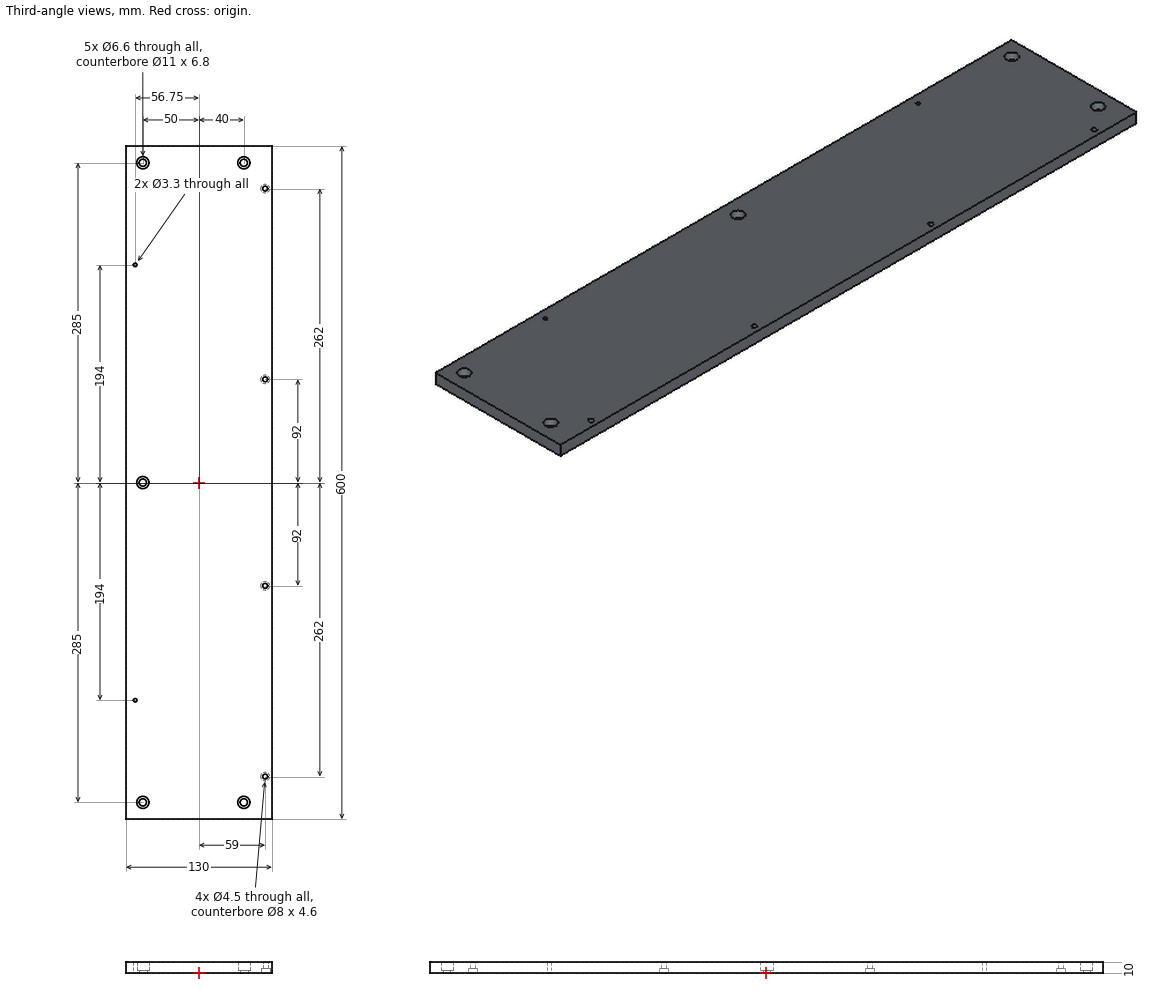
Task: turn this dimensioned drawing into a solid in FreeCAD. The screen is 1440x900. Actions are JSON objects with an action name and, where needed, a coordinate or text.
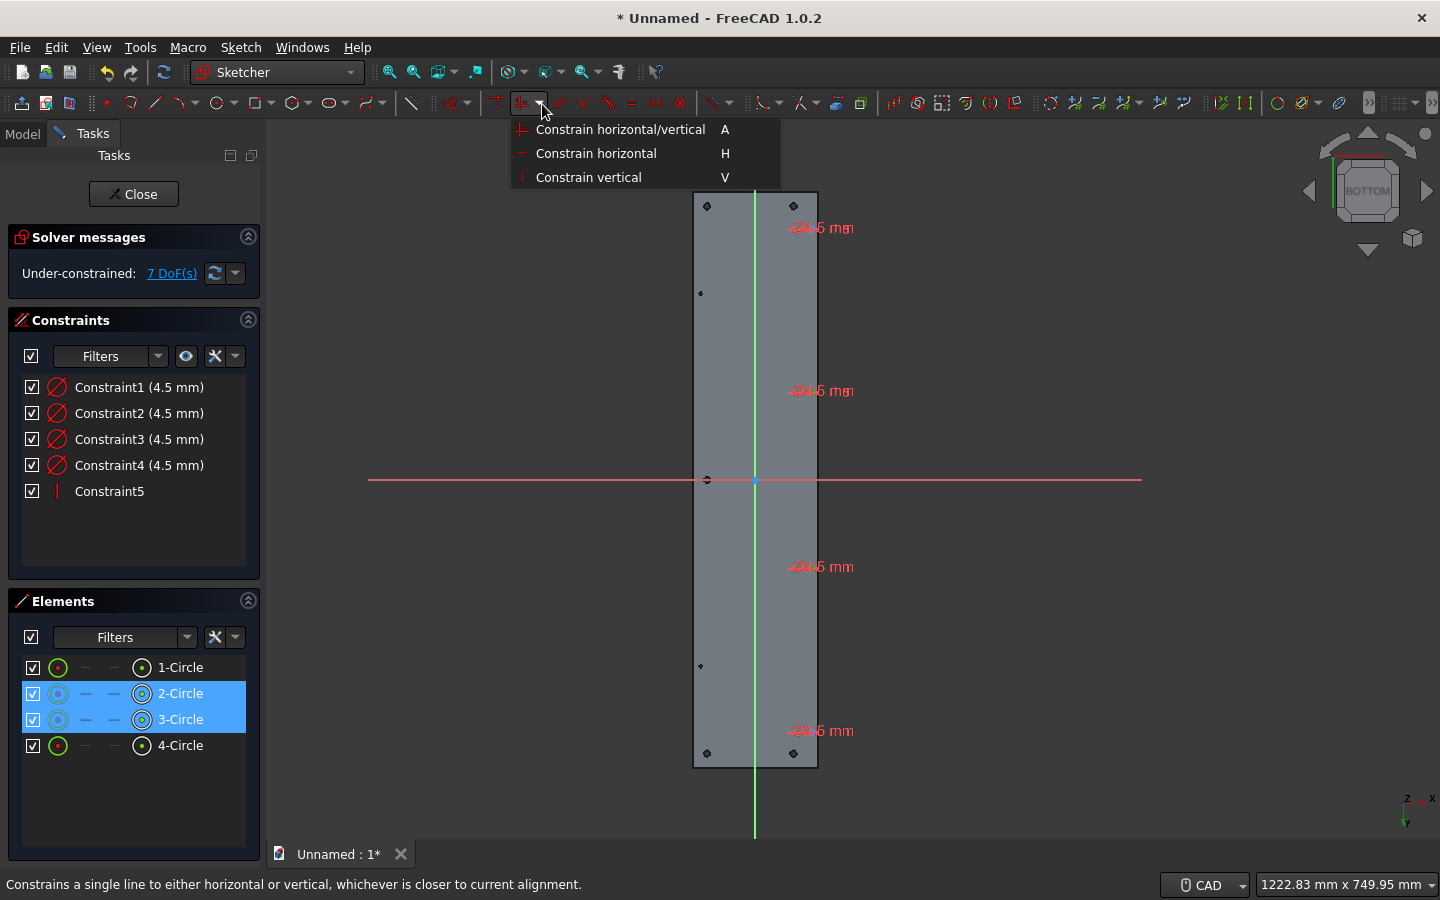
{"action": "left_click", "coordinate": [646, 177]}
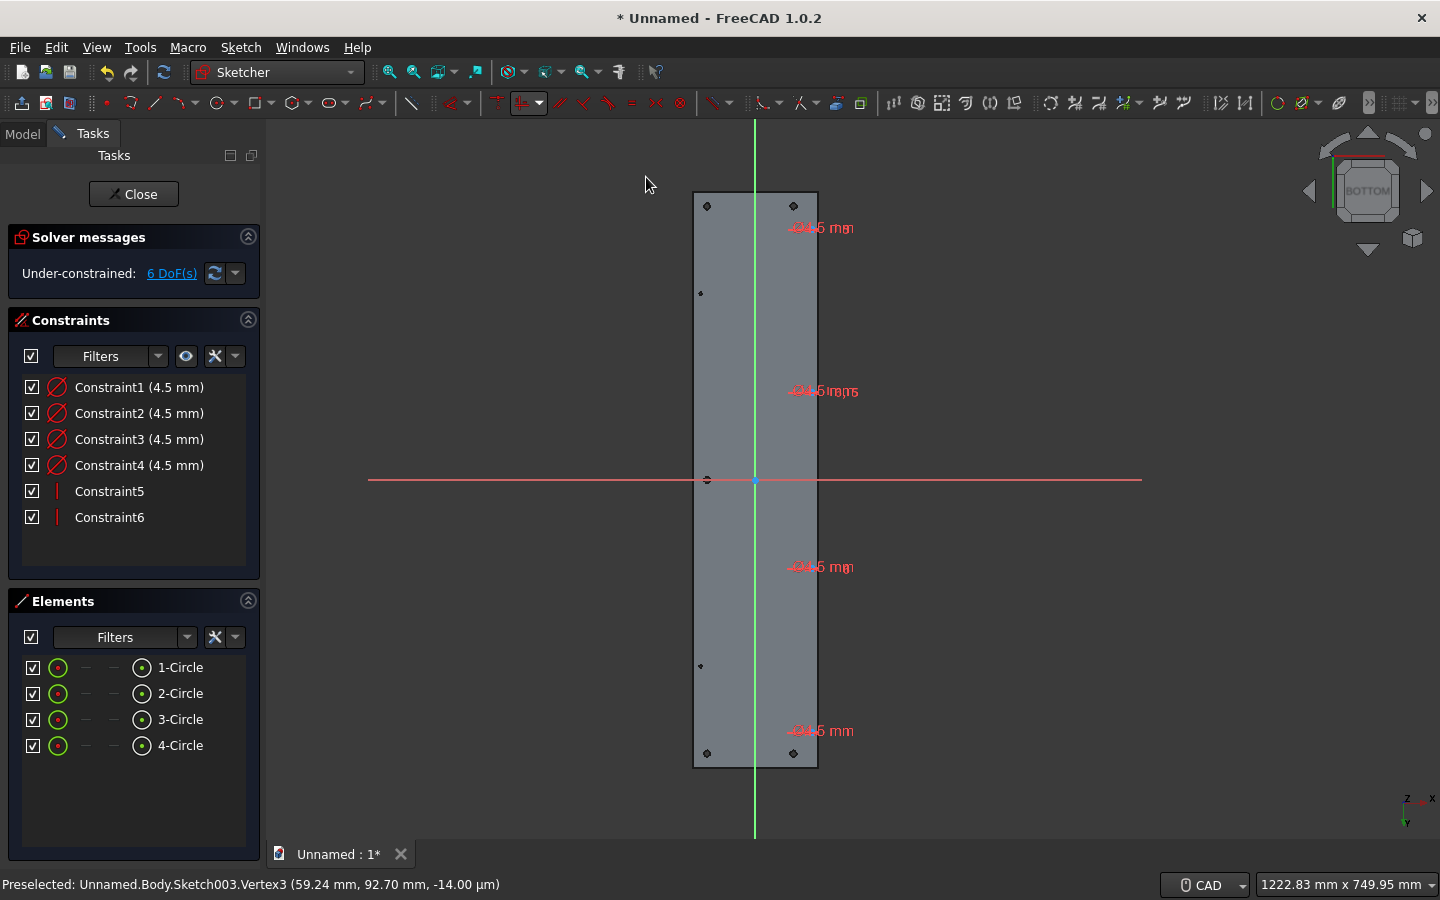
{"action": "left_click", "coordinate": [812, 569]}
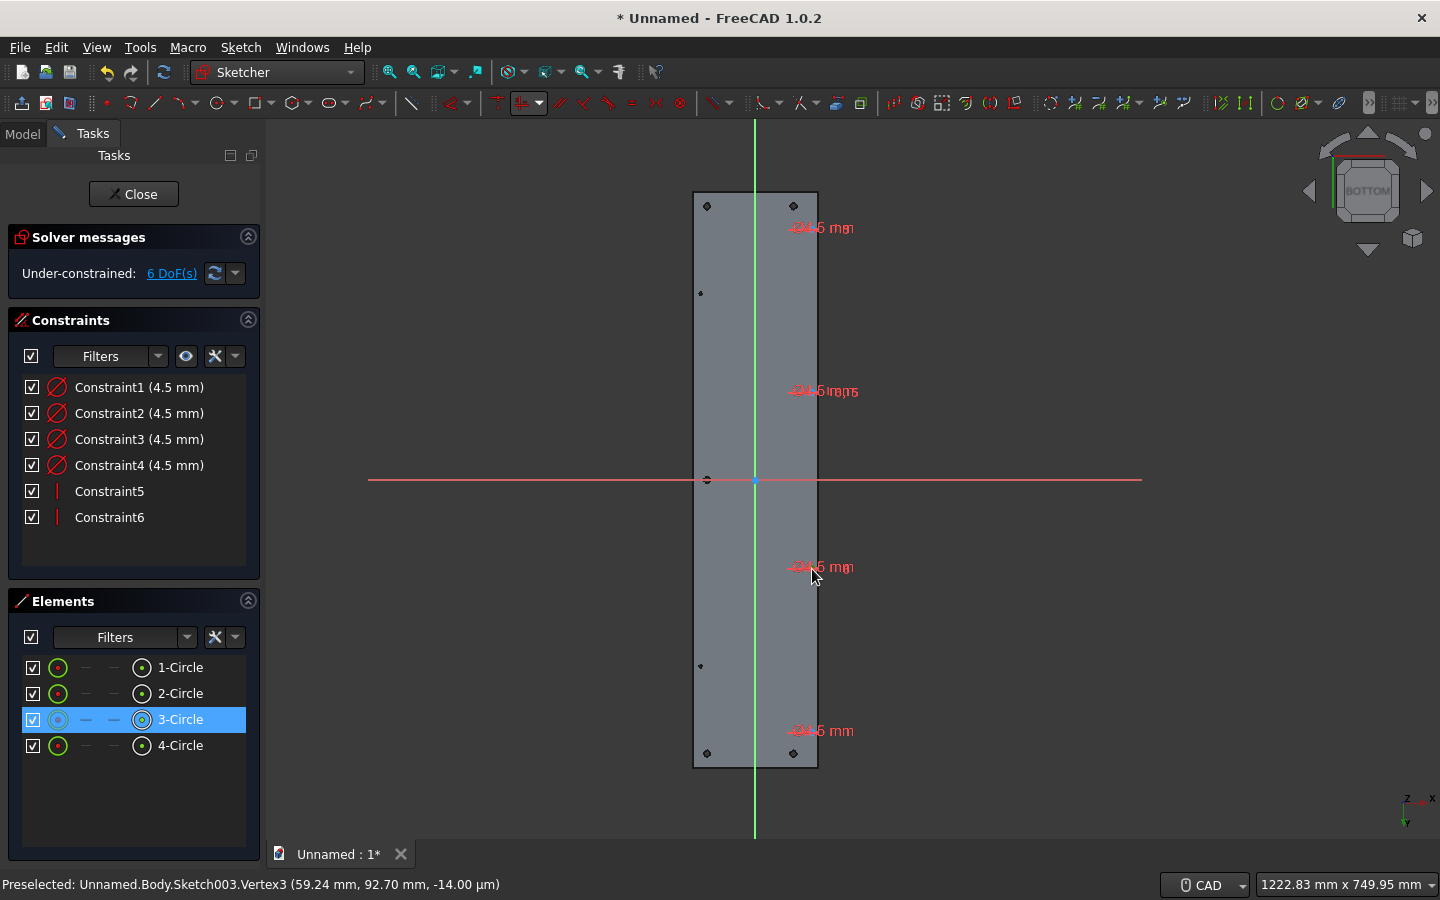
{"action": "left_click", "coordinate": [812, 733]}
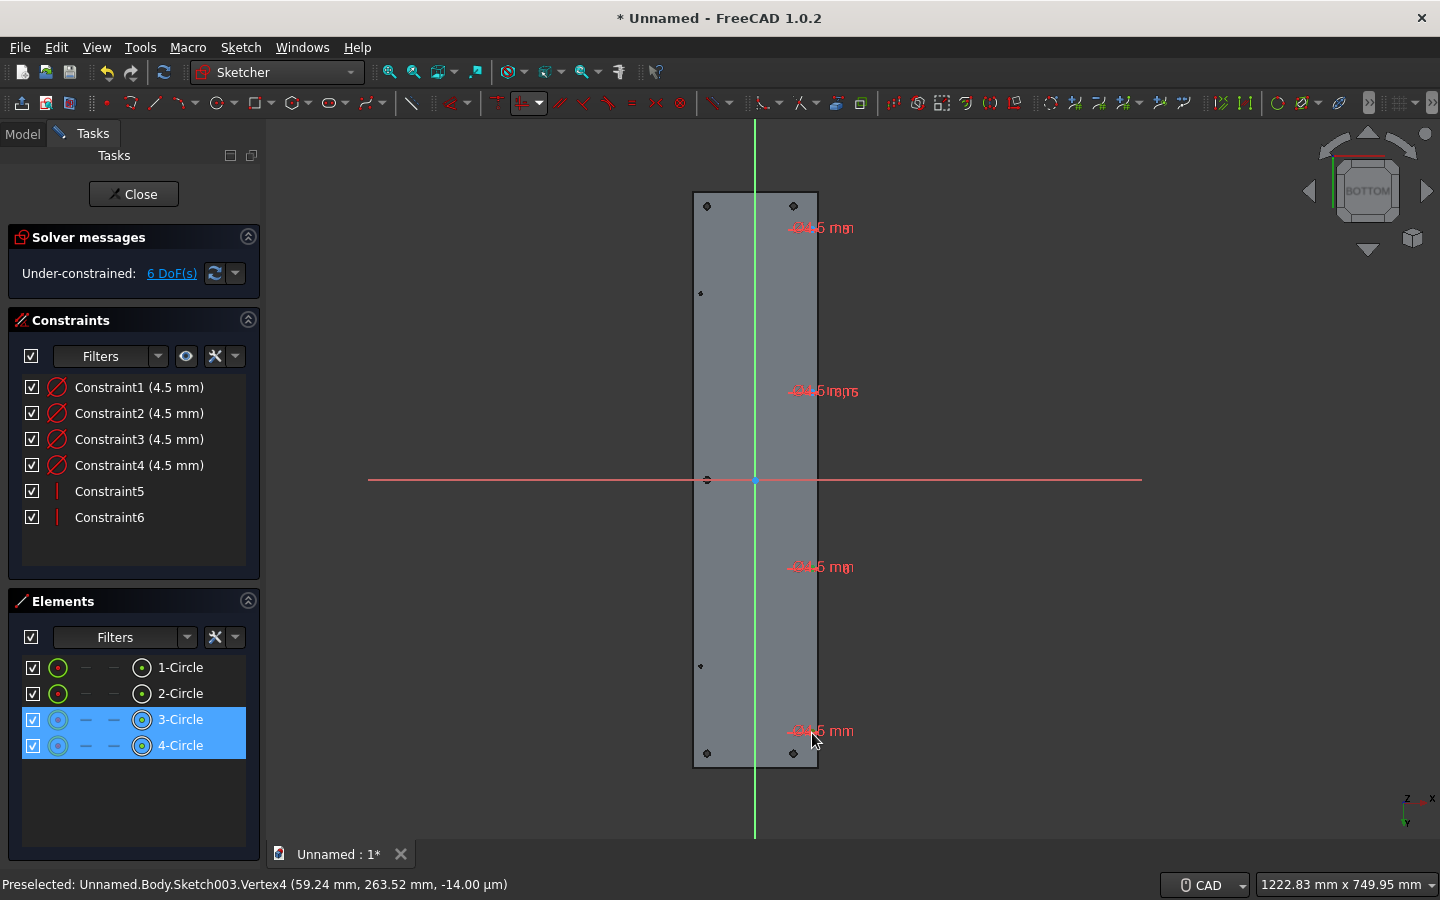
{"action": "key", "text": "v"}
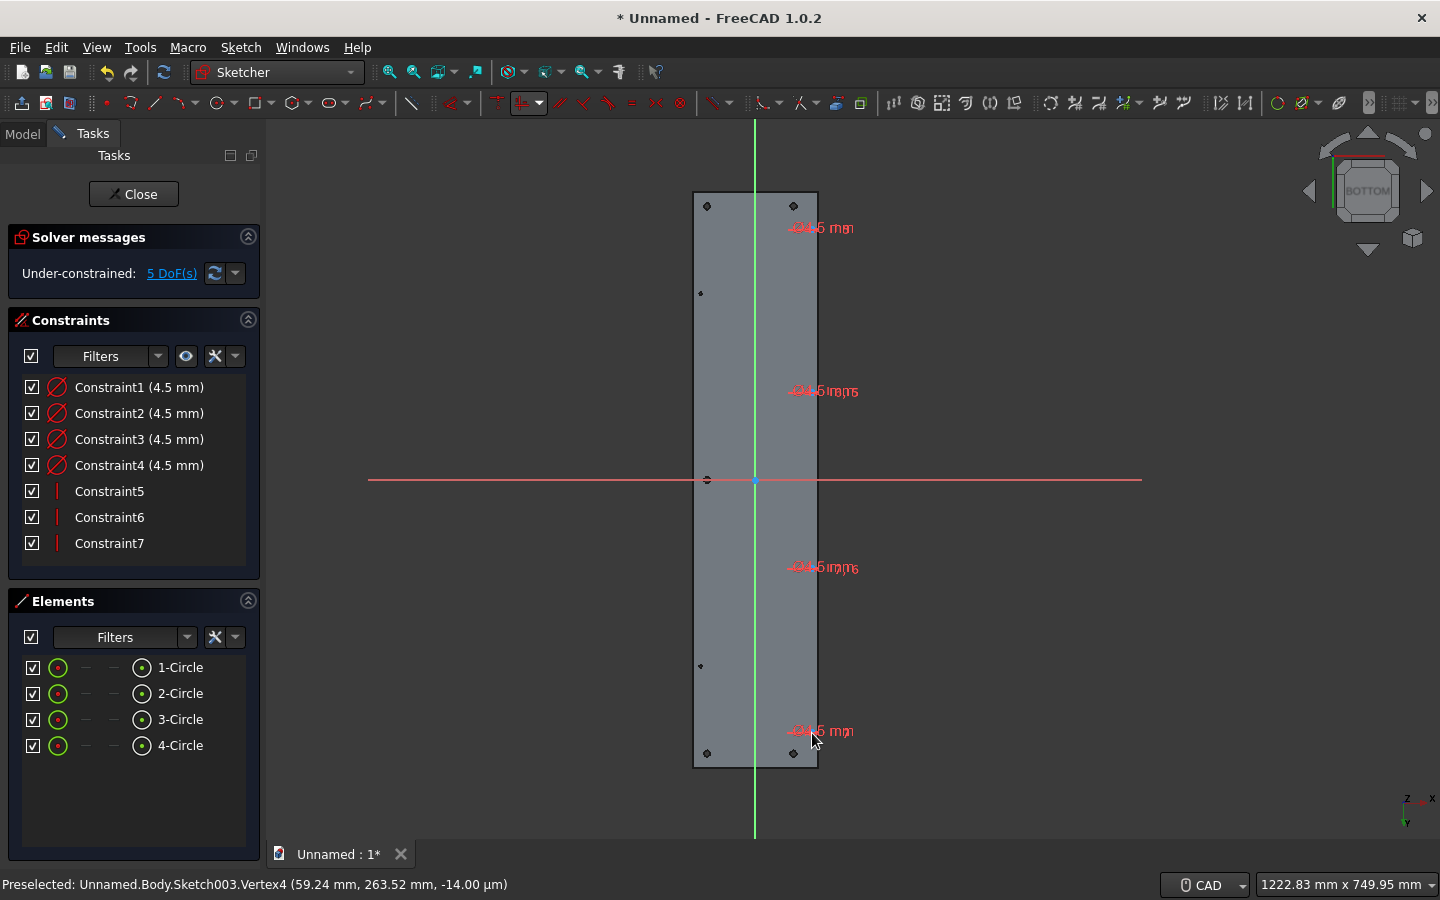
{"action": "key", "text": "d"}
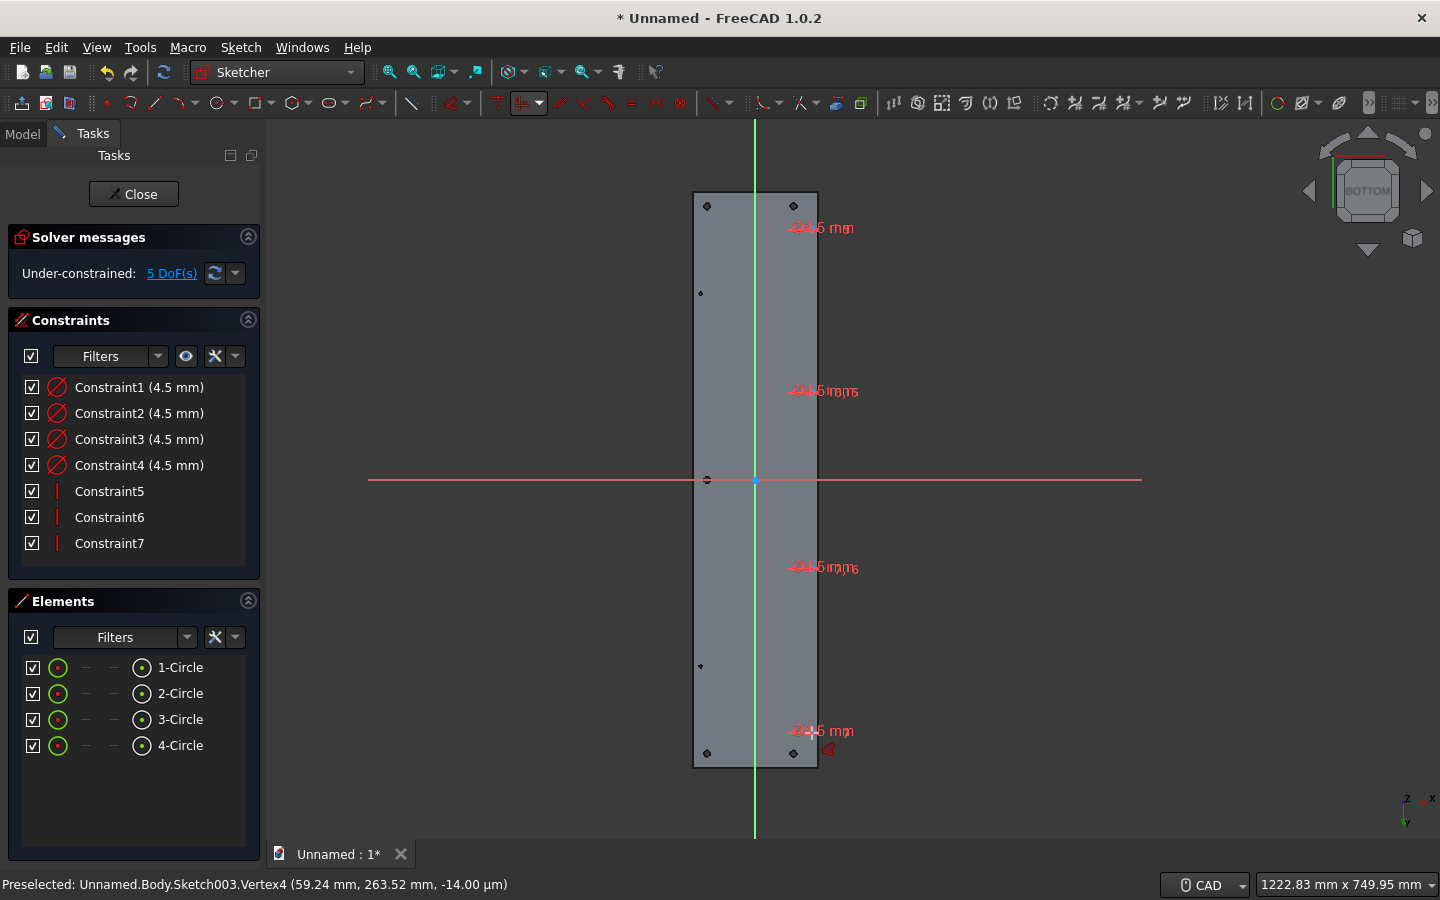
{"action": "left_click", "coordinate": [812, 230]}
{"action": "left_click", "coordinate": [784, 196]}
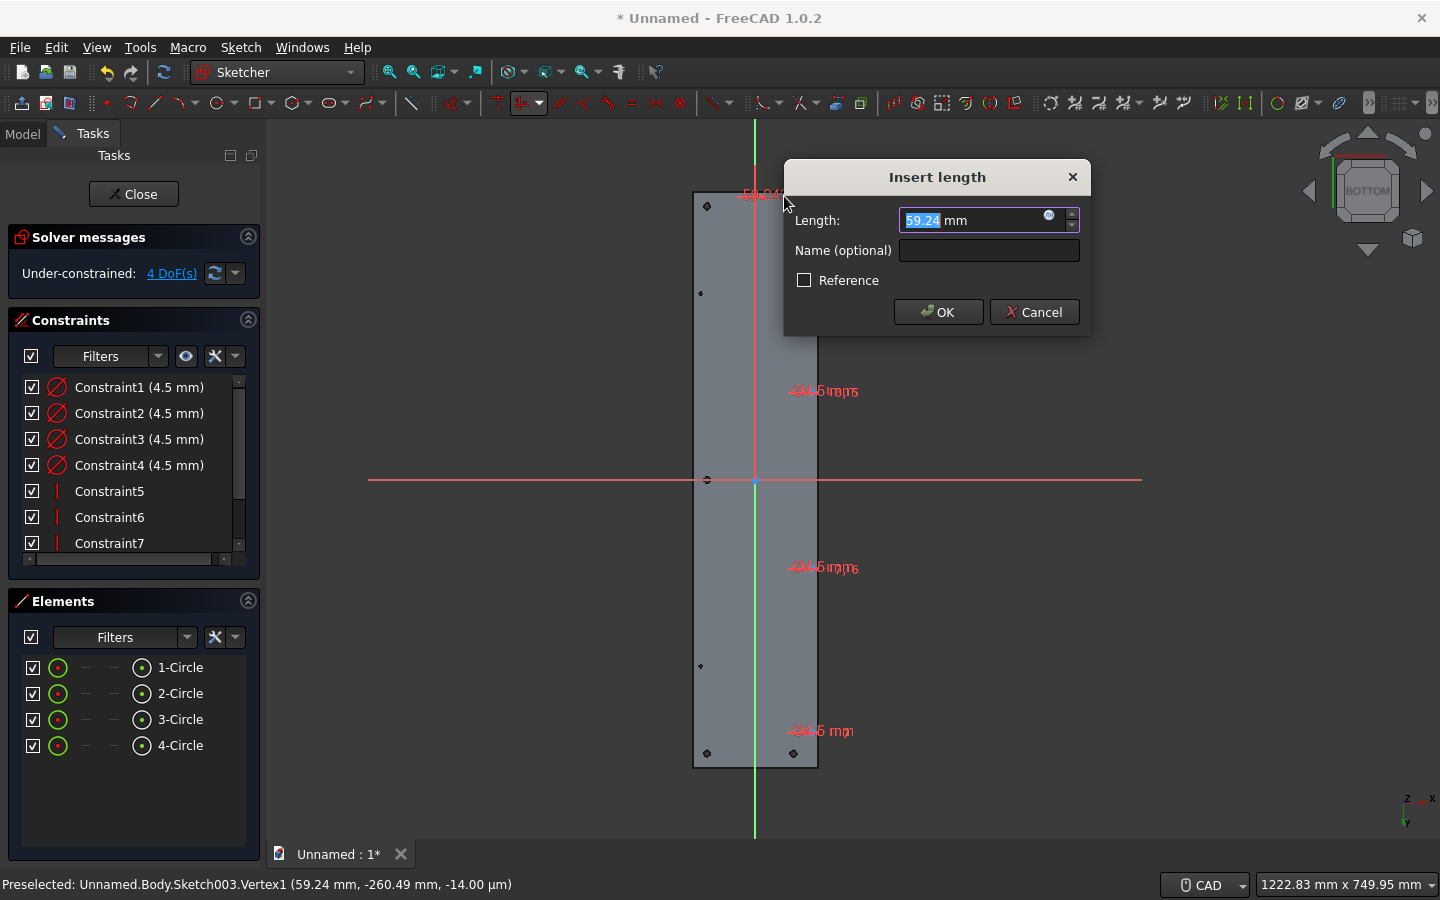
{"action": "type", "text": "59"}
{"action": "key", "text": "Return"}